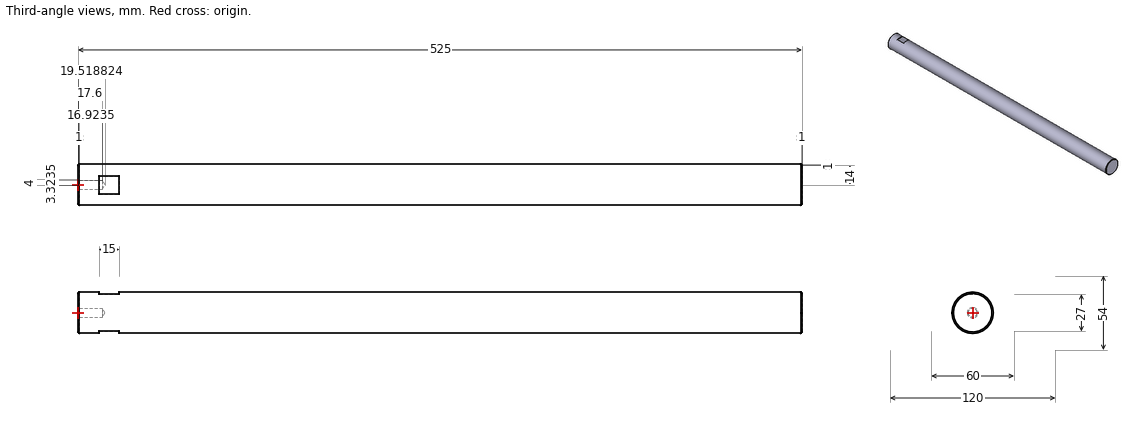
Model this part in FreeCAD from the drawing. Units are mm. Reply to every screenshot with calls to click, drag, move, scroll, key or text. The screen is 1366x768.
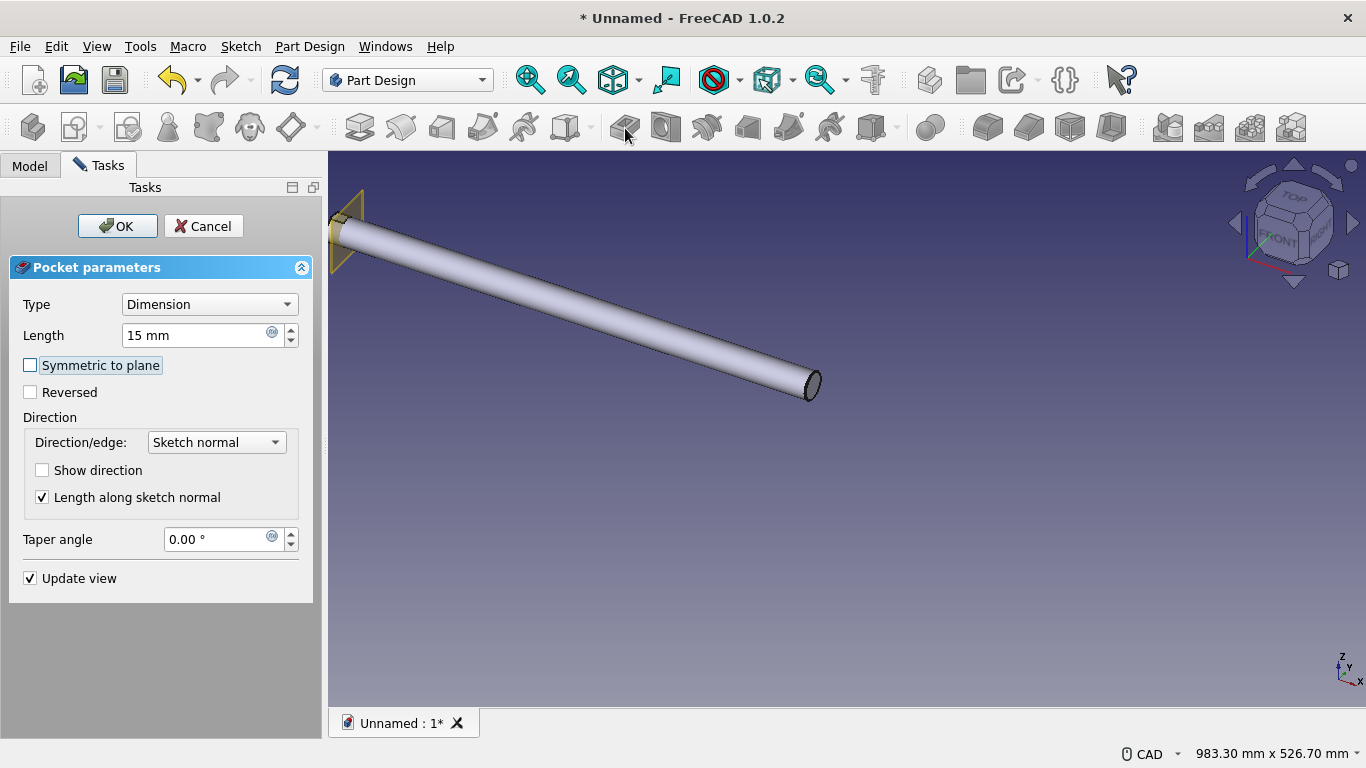
click(31, 392)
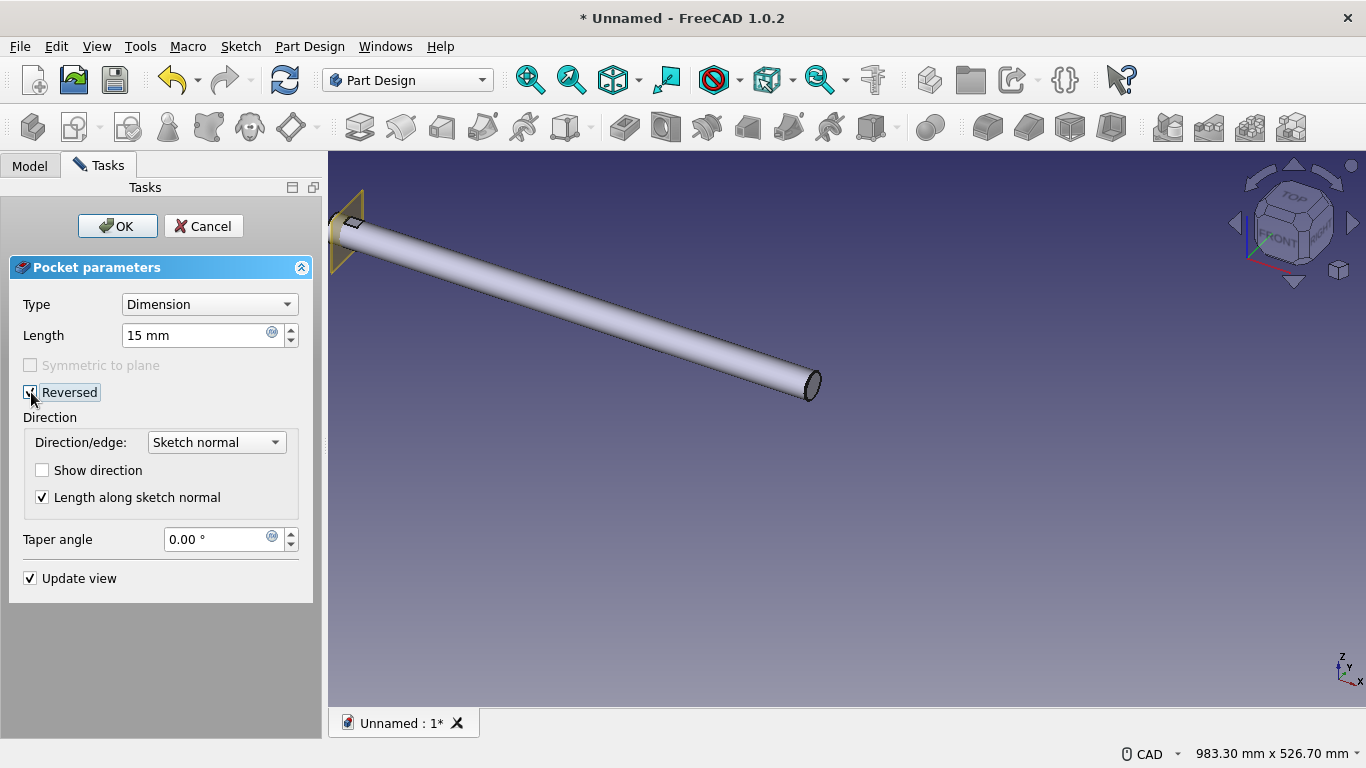
click(118, 226)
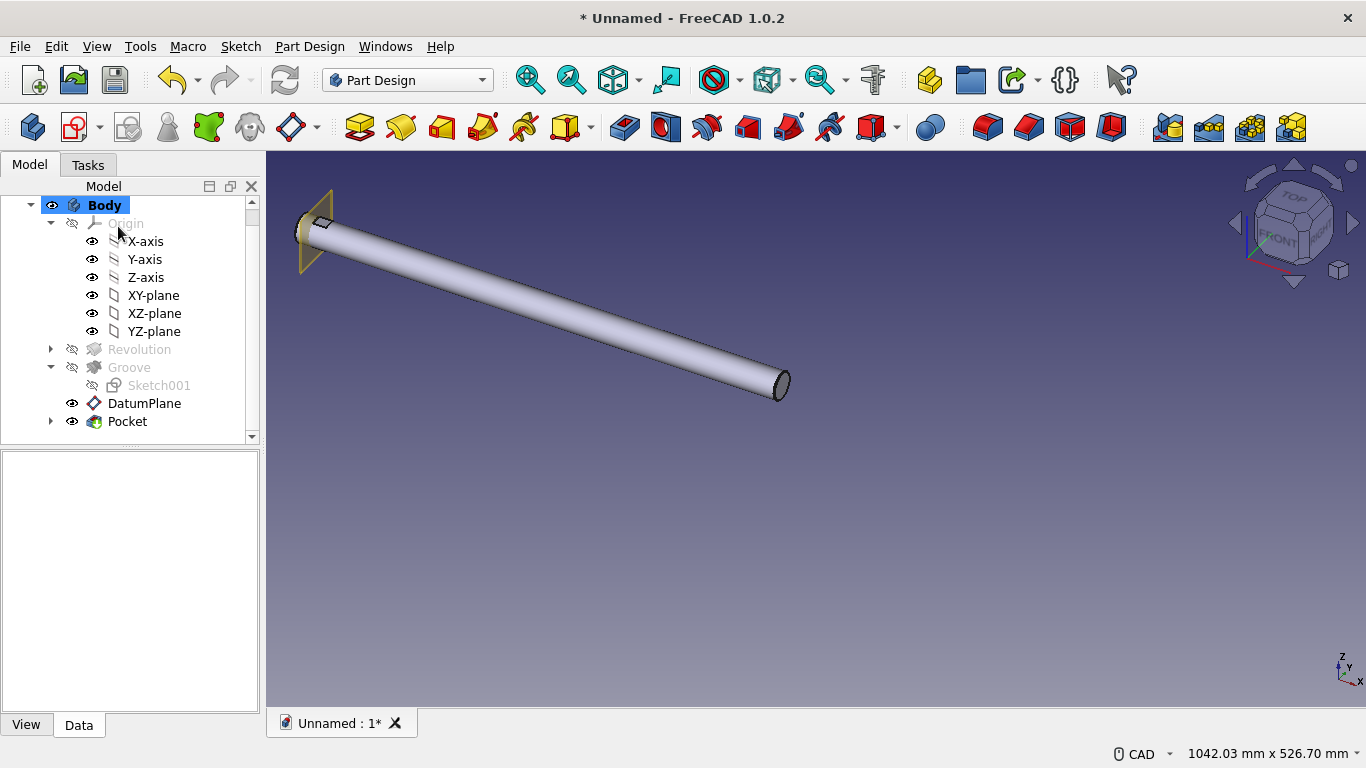
click(117, 403)
key(space)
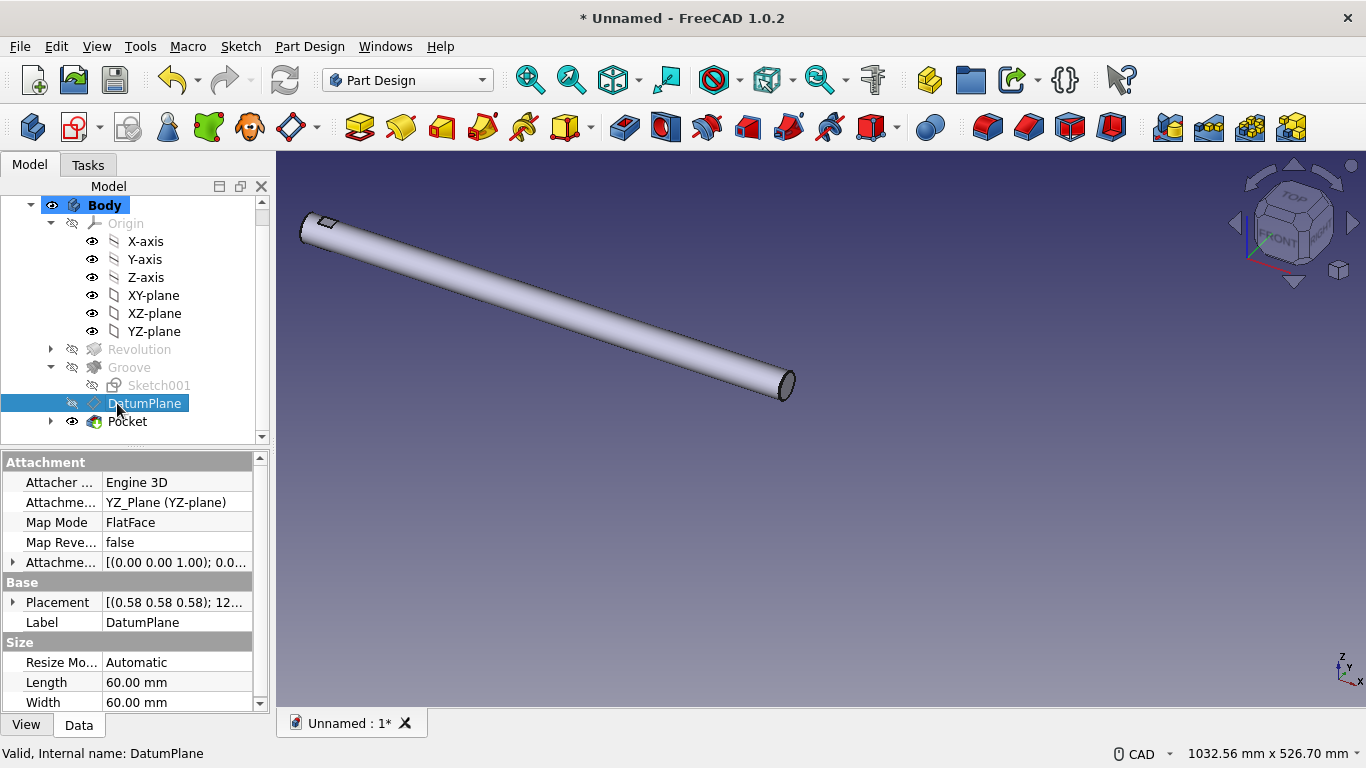
key(0)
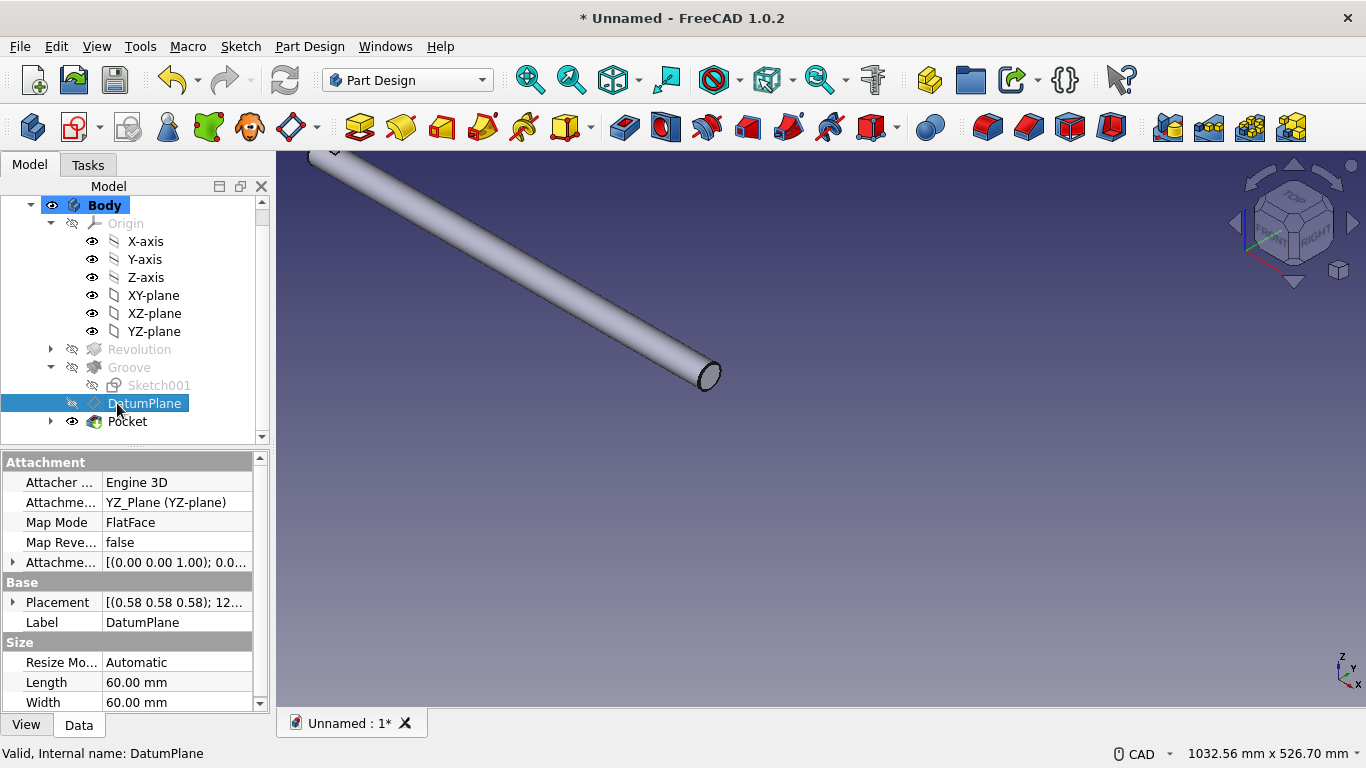
click(531, 80)